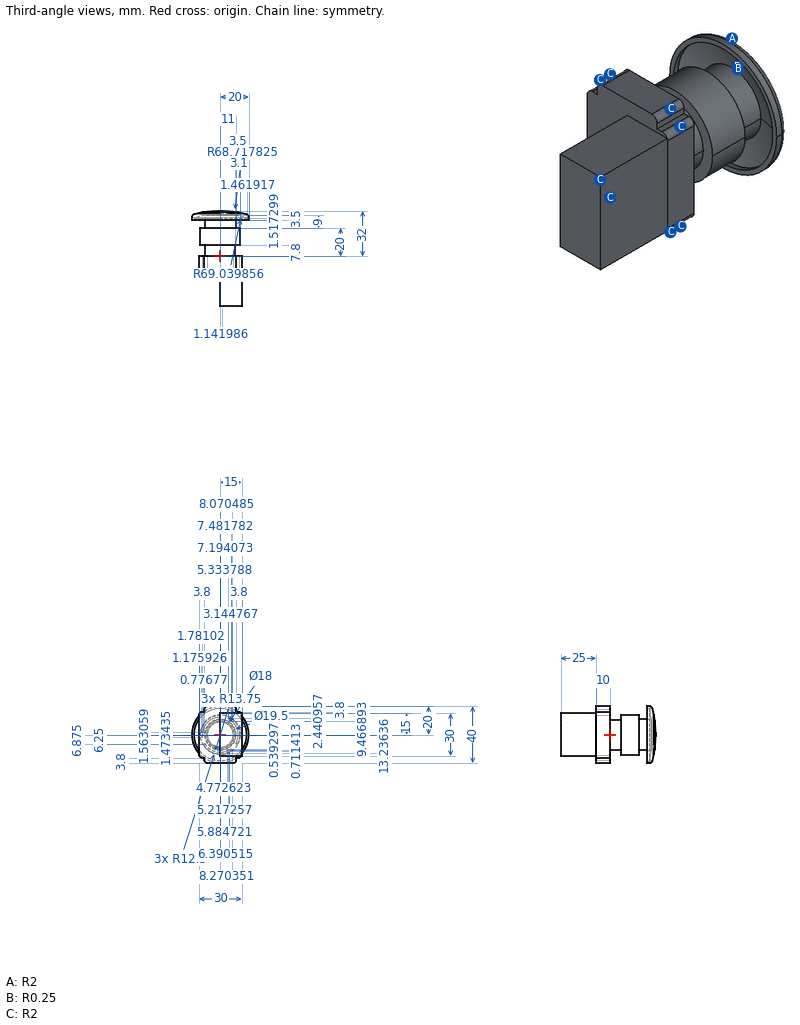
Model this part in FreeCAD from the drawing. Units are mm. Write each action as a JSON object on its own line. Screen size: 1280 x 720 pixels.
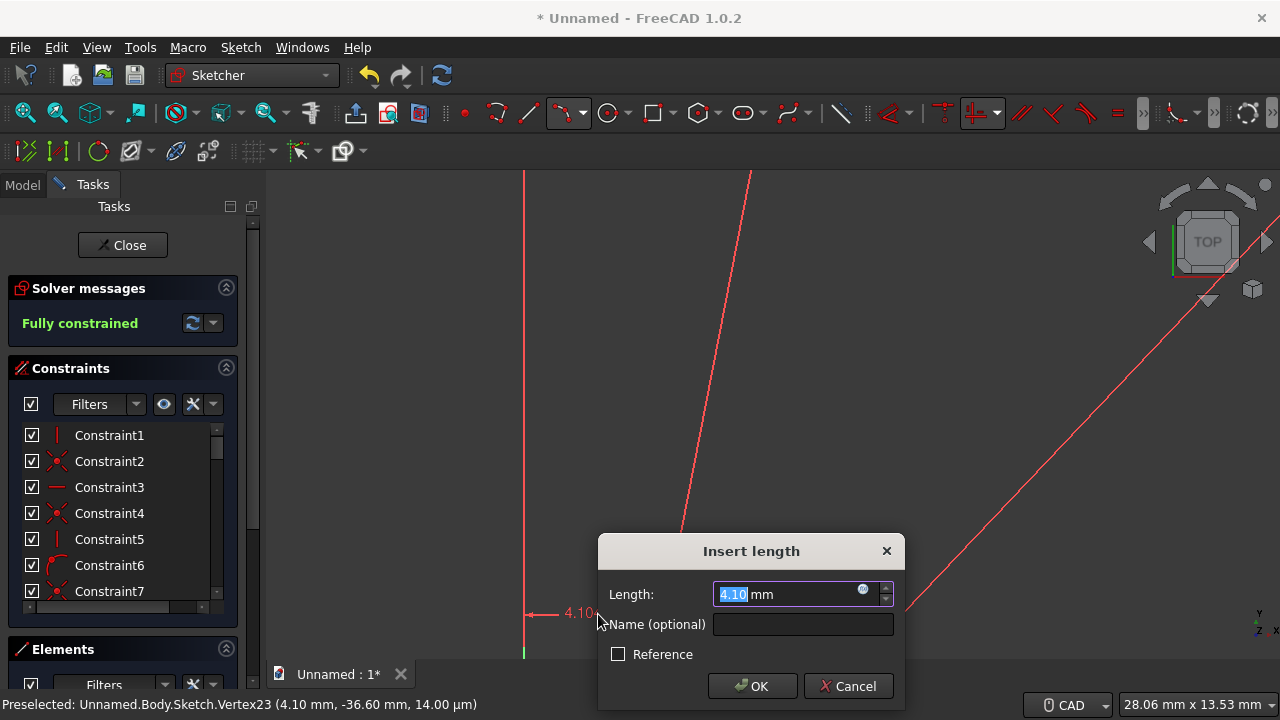
{"action": "type", "text": "1.141986"}
{"action": "key", "text": "Return"}
{"action": "key", "text": "Escape"}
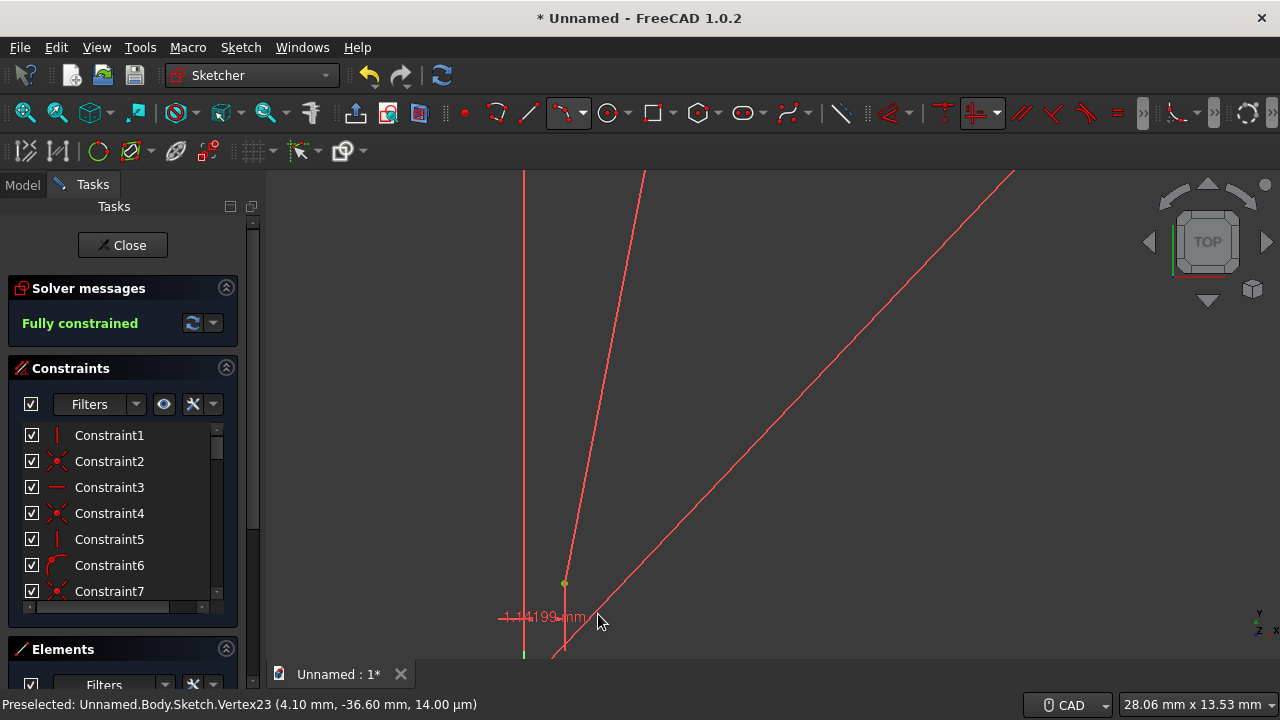
{"action": "left_click", "coordinate": [123, 245]}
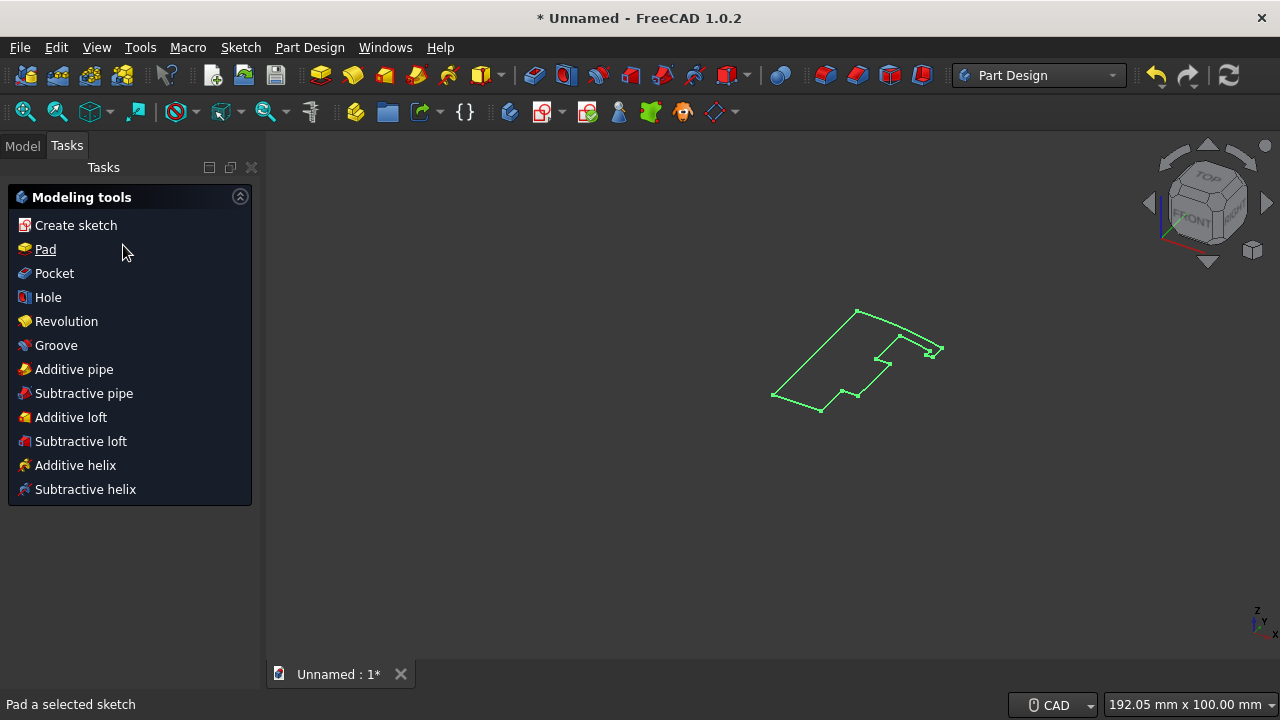
{"action": "left_click", "coordinate": [354, 76]}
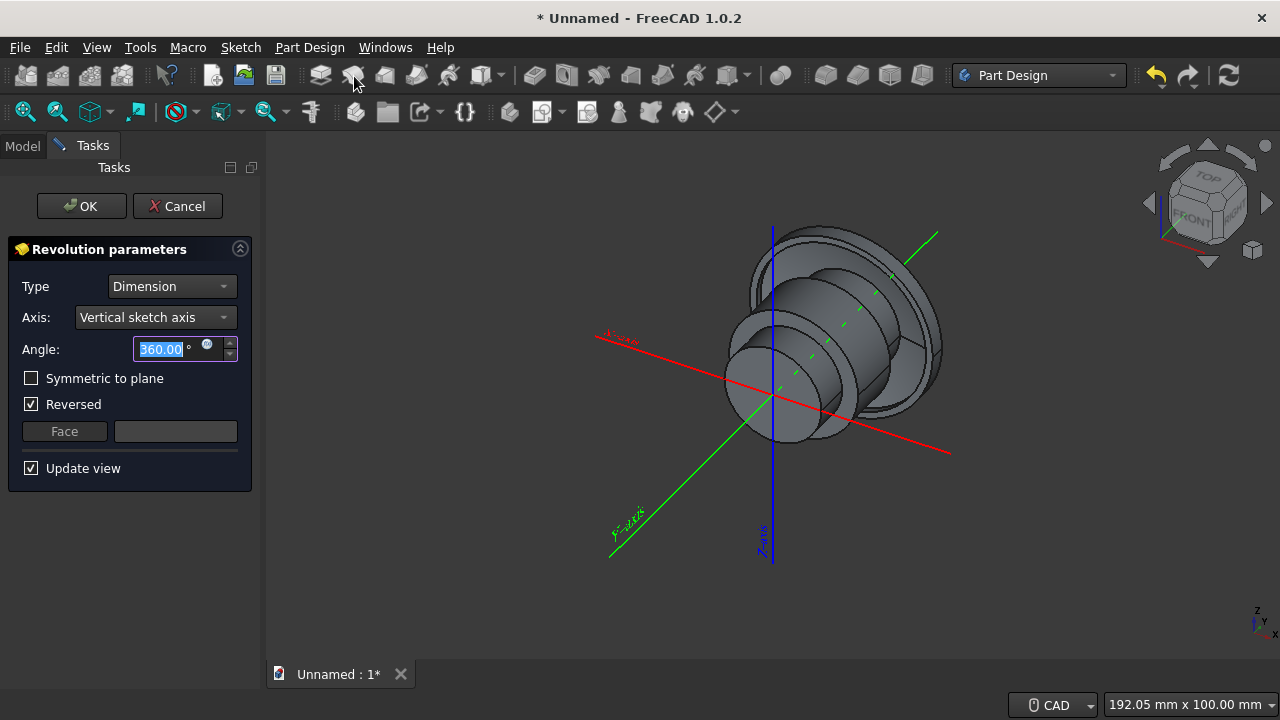
{"action": "left_click", "coordinate": [82, 206]}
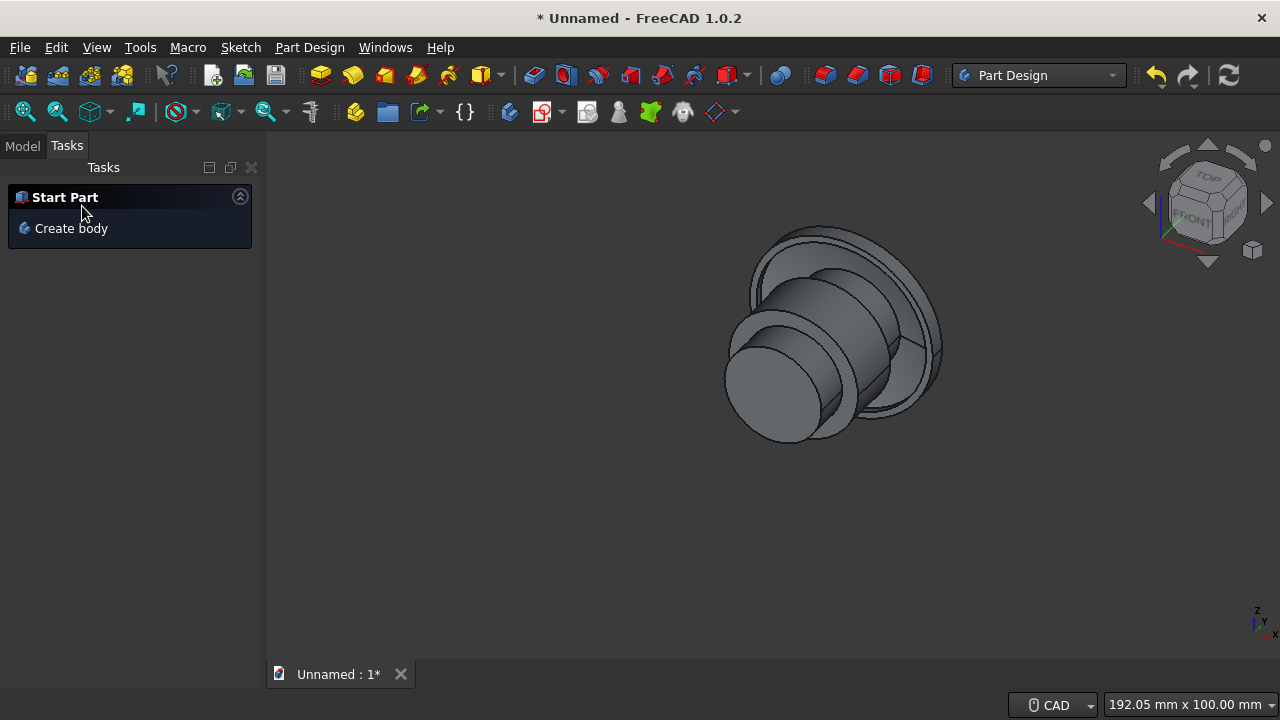
{"action": "key", "text": "0"}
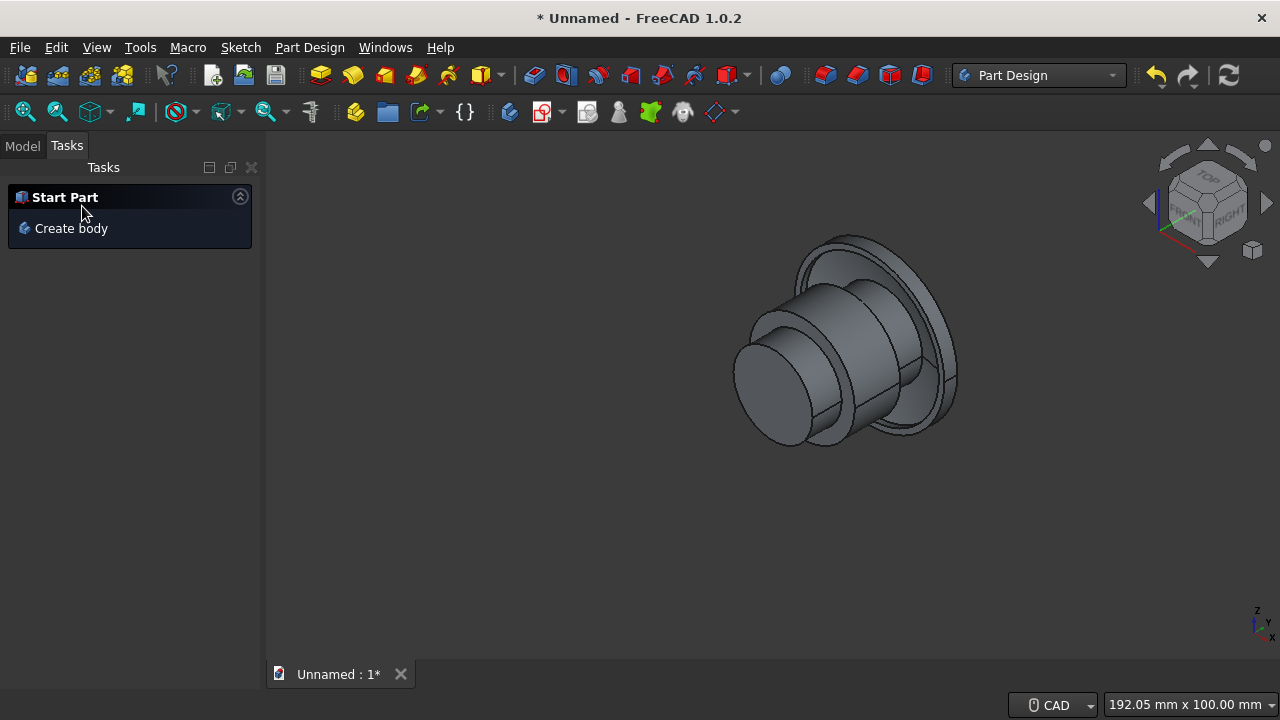
{"action": "left_click", "coordinate": [906, 262]}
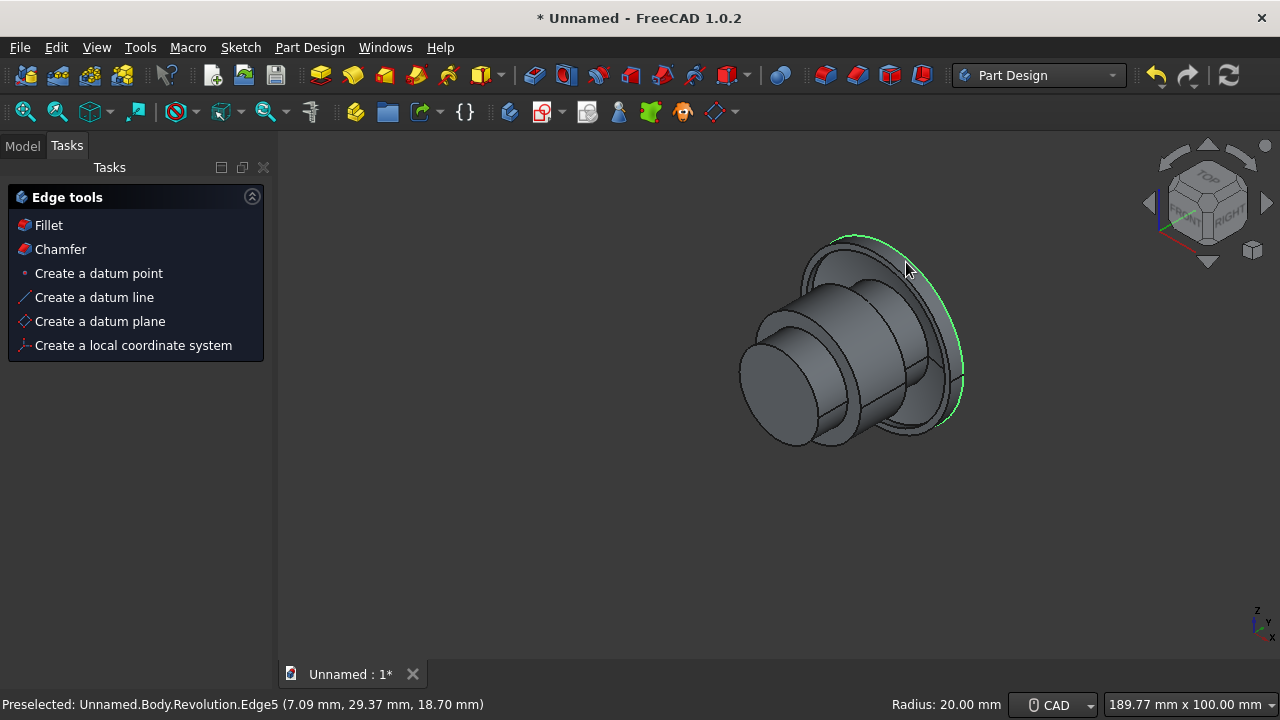
{"action": "left_click", "coordinate": [826, 76]}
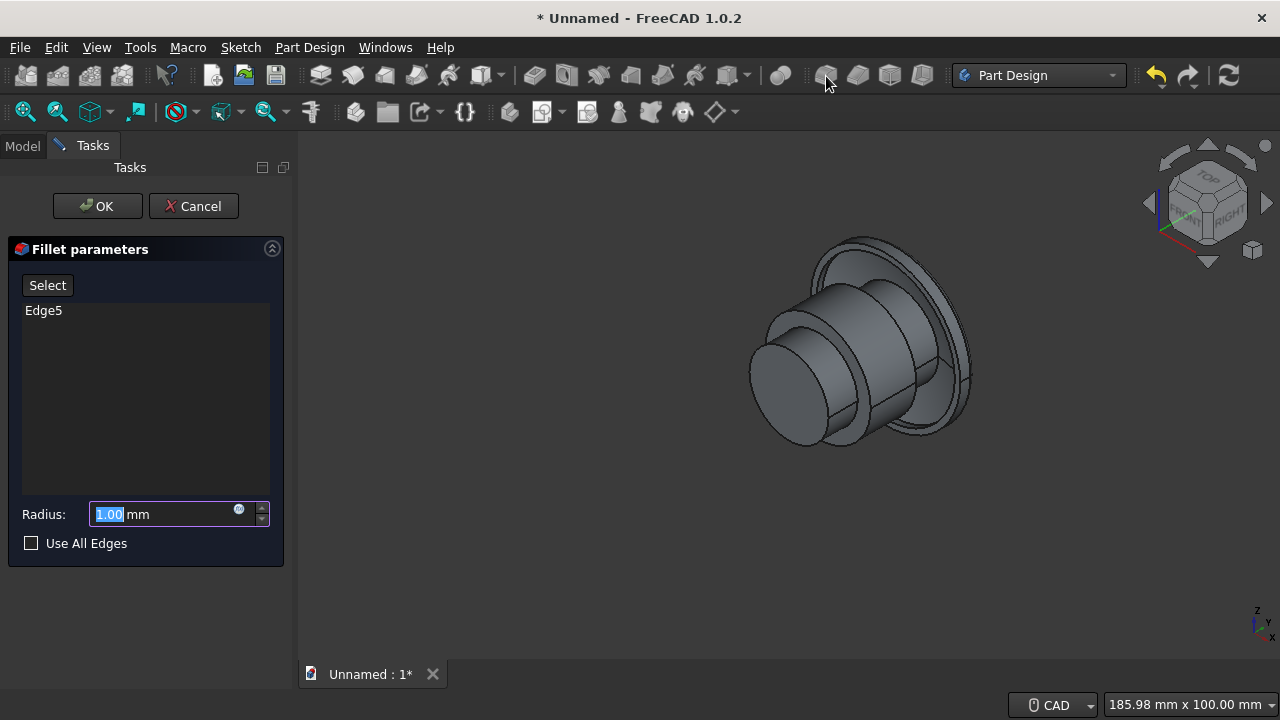
{"action": "type", "text": "2"}
{"action": "key", "text": "Tab"}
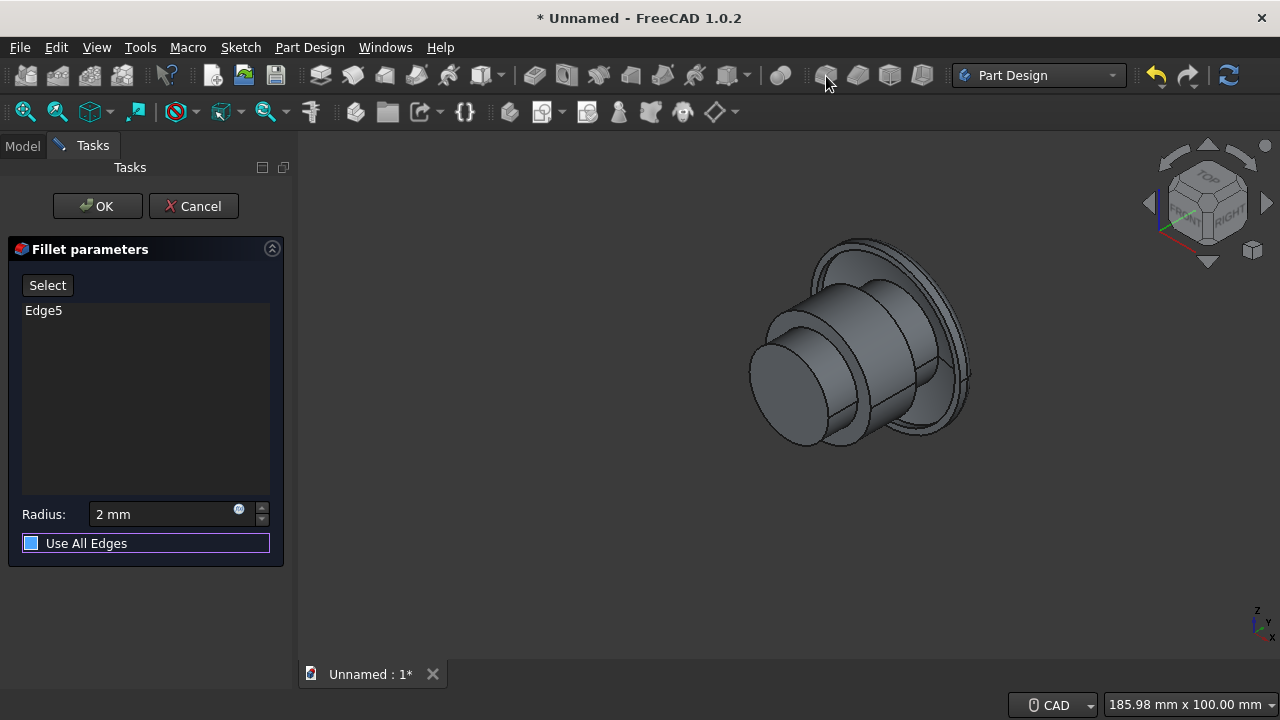
{"action": "left_click", "coordinate": [98, 206]}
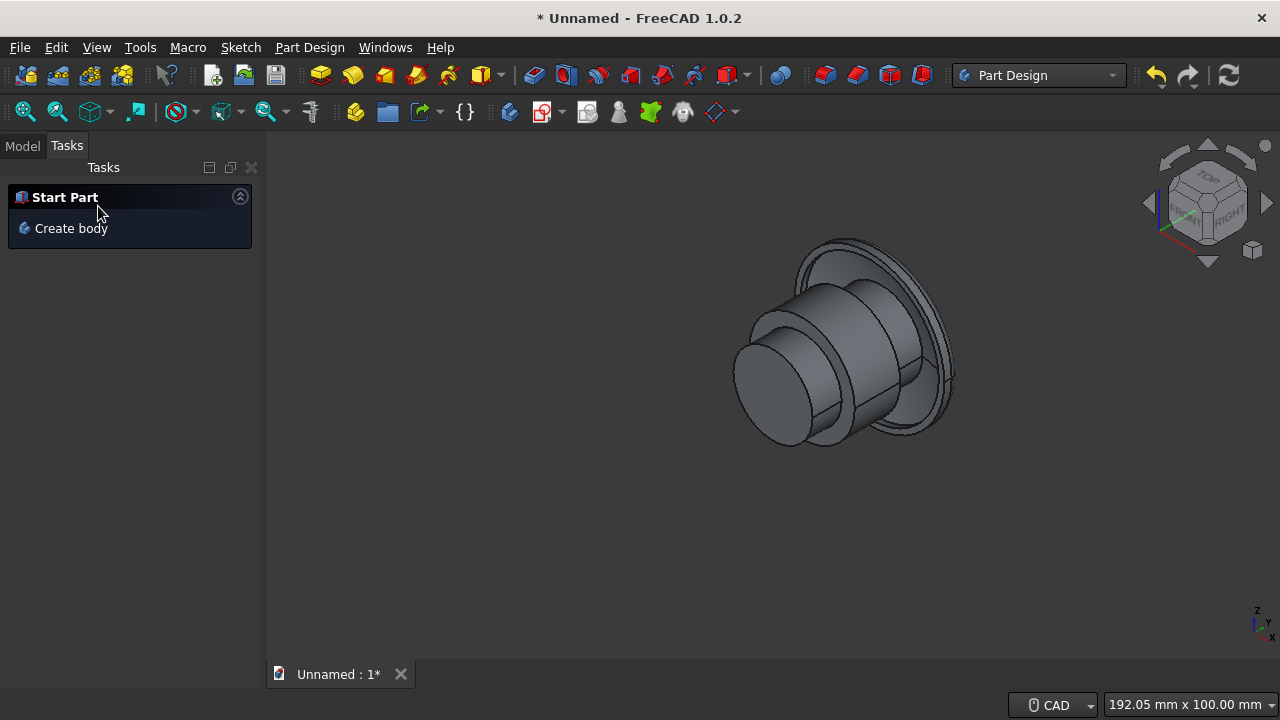
{"action": "left_click", "coordinate": [23, 145]}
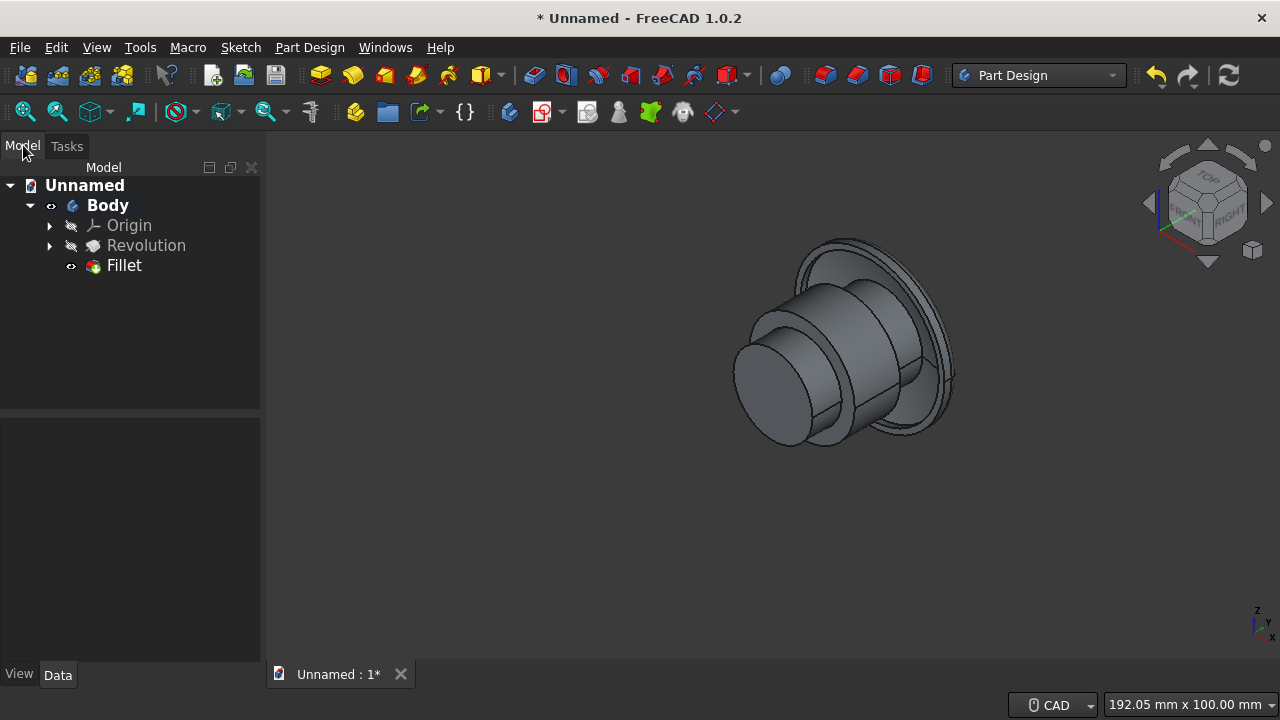
{"action": "left_click", "coordinate": [50, 226]}